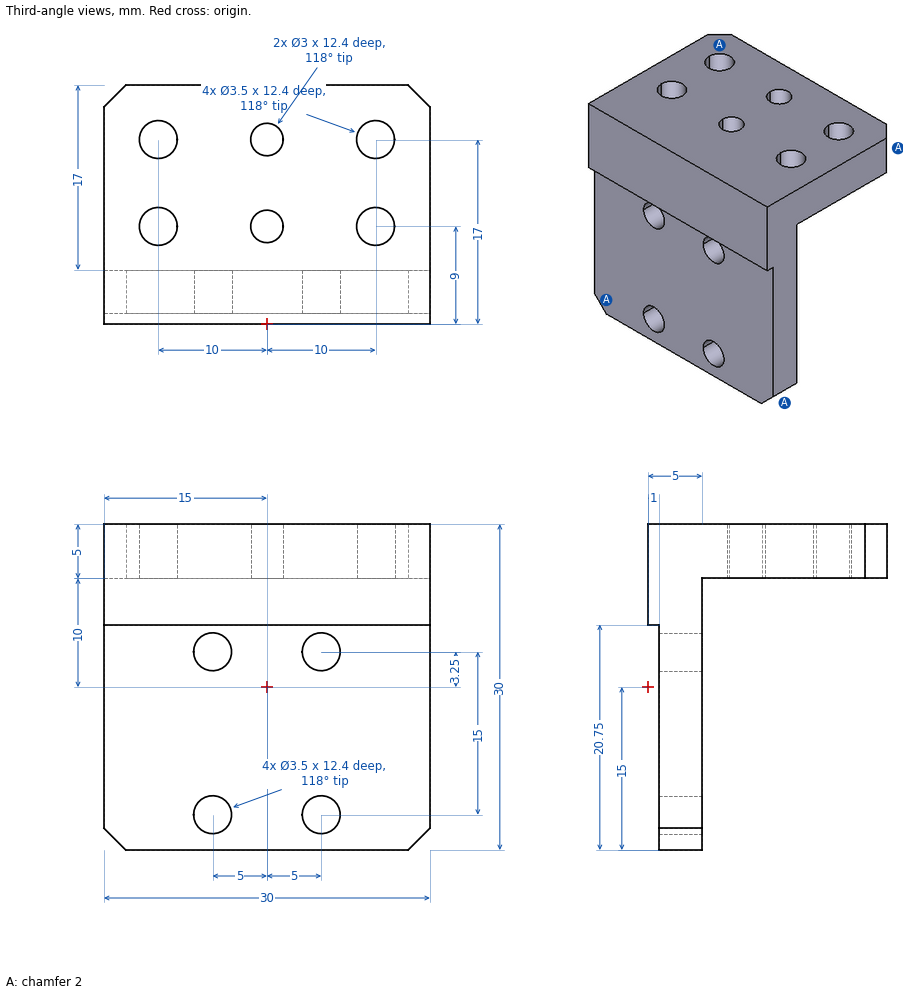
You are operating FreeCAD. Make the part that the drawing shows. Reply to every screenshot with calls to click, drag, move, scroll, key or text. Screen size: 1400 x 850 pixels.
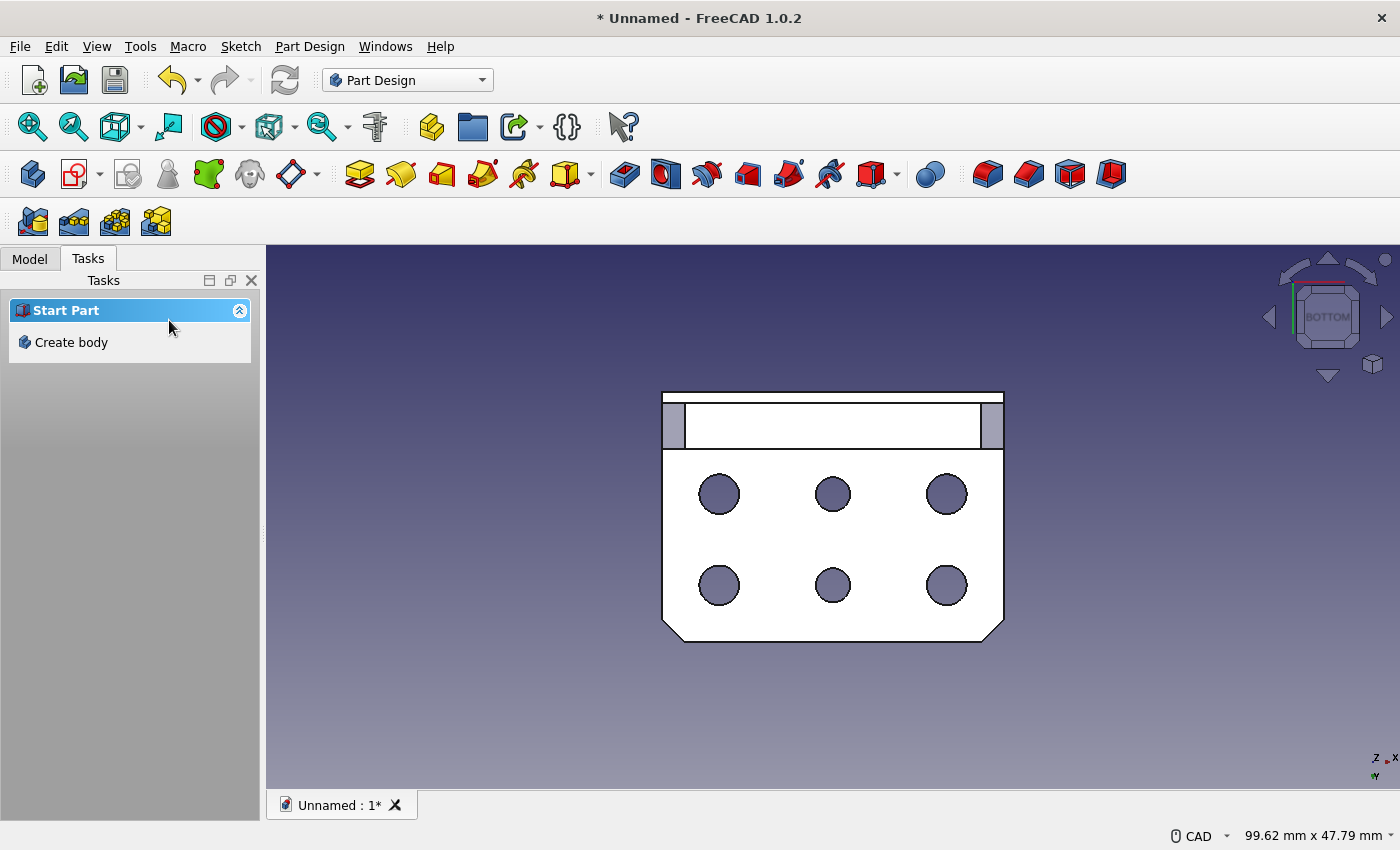
key(0)